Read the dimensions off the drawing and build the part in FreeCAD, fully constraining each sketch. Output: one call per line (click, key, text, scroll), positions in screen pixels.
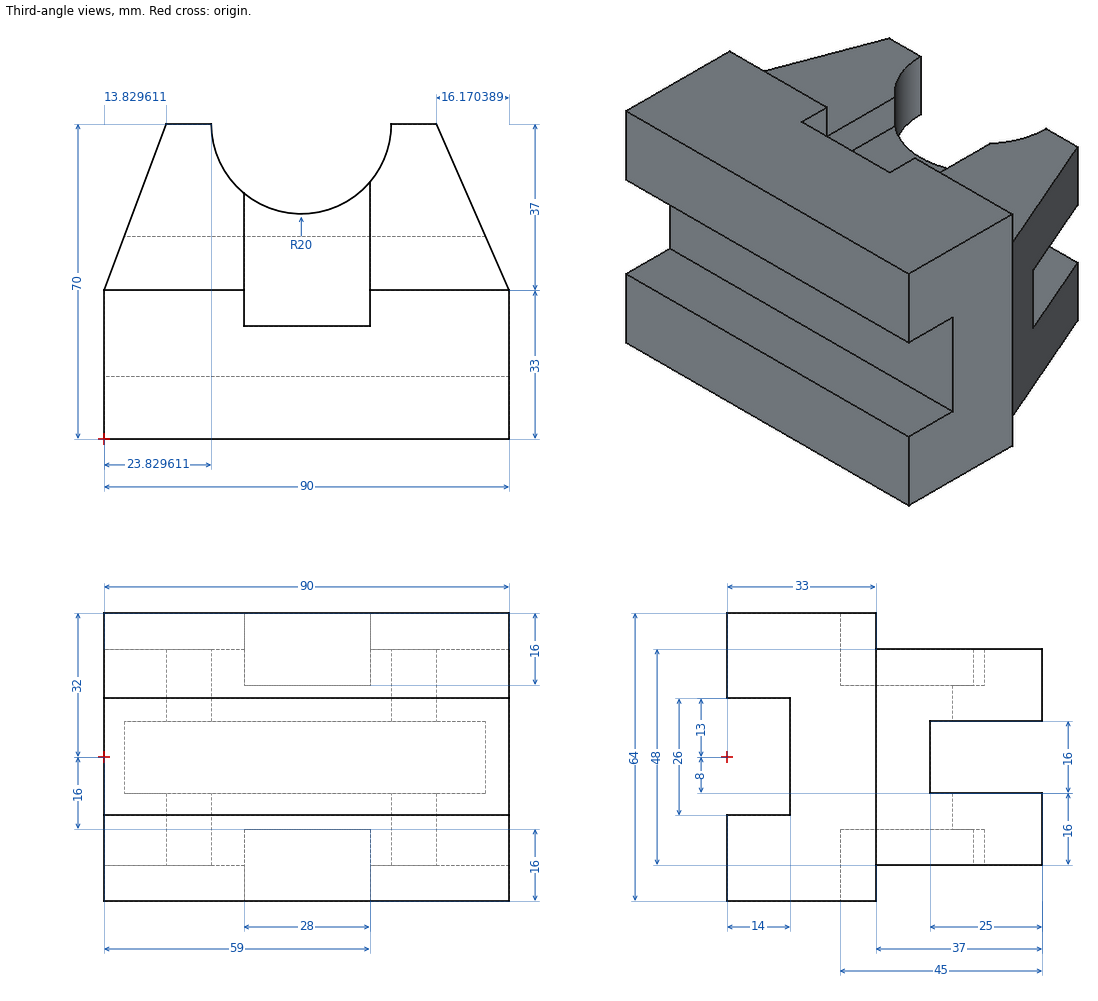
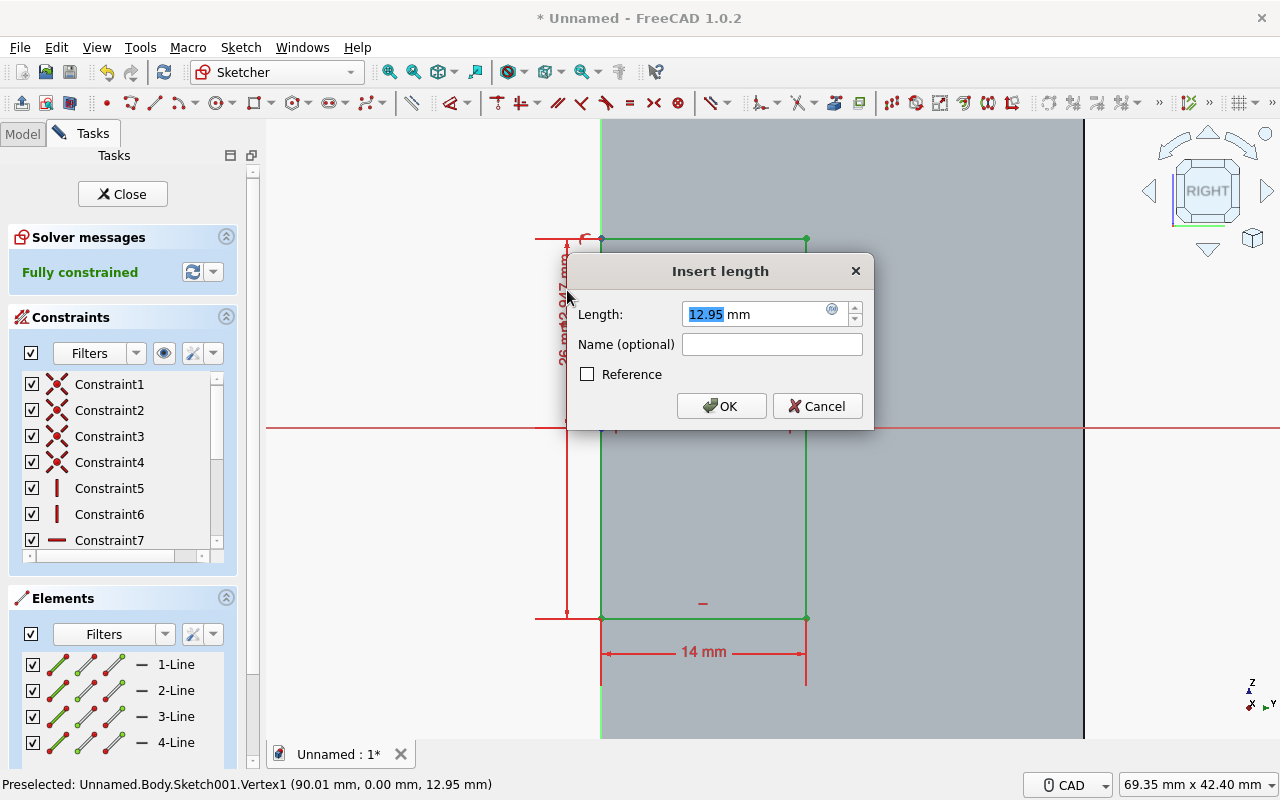
text(13)
key(Return)
key(Escape)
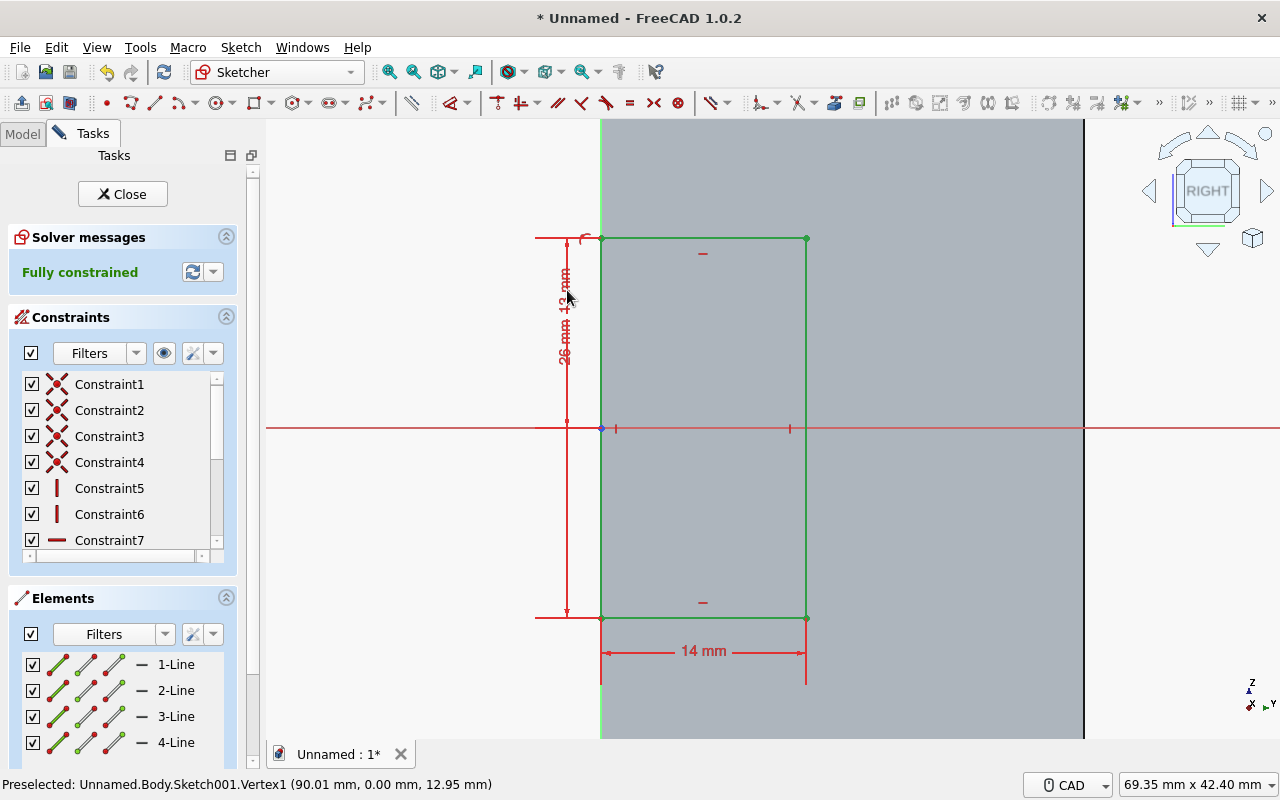
click(123, 194)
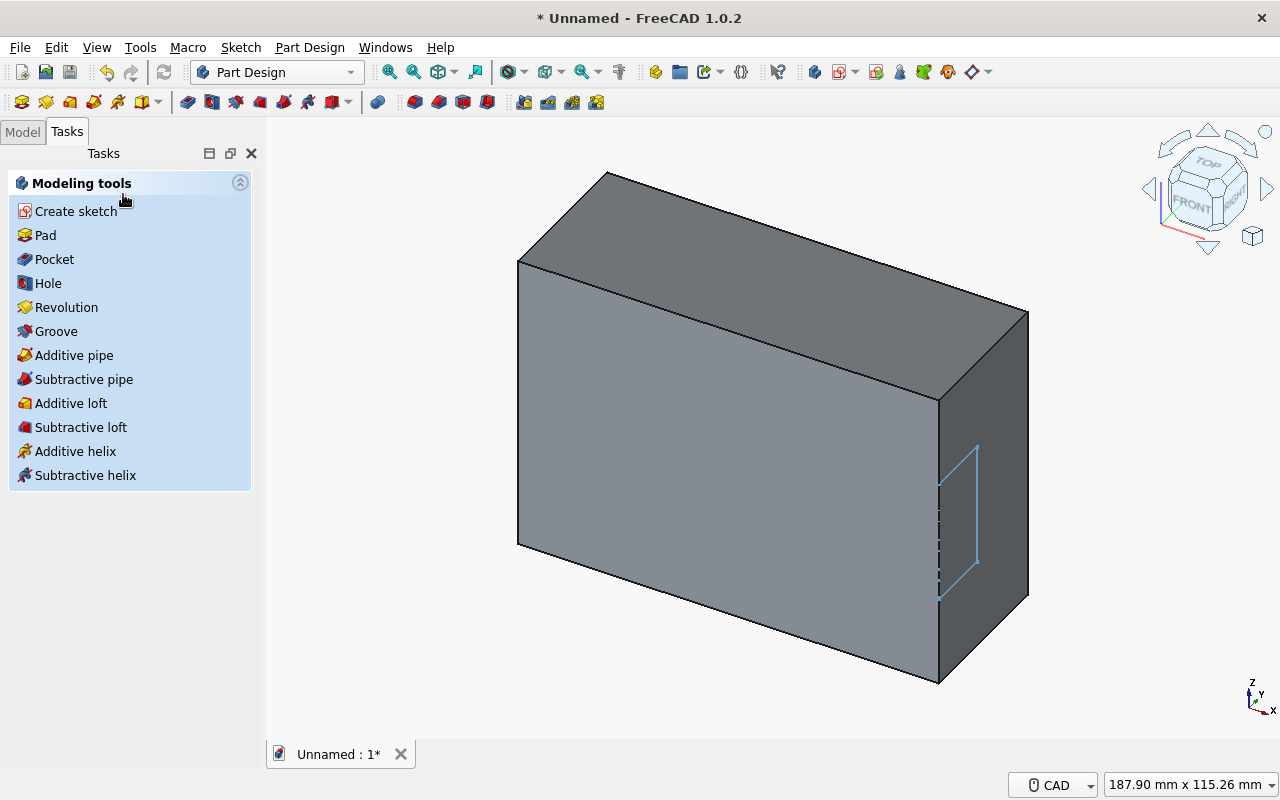
click(188, 102)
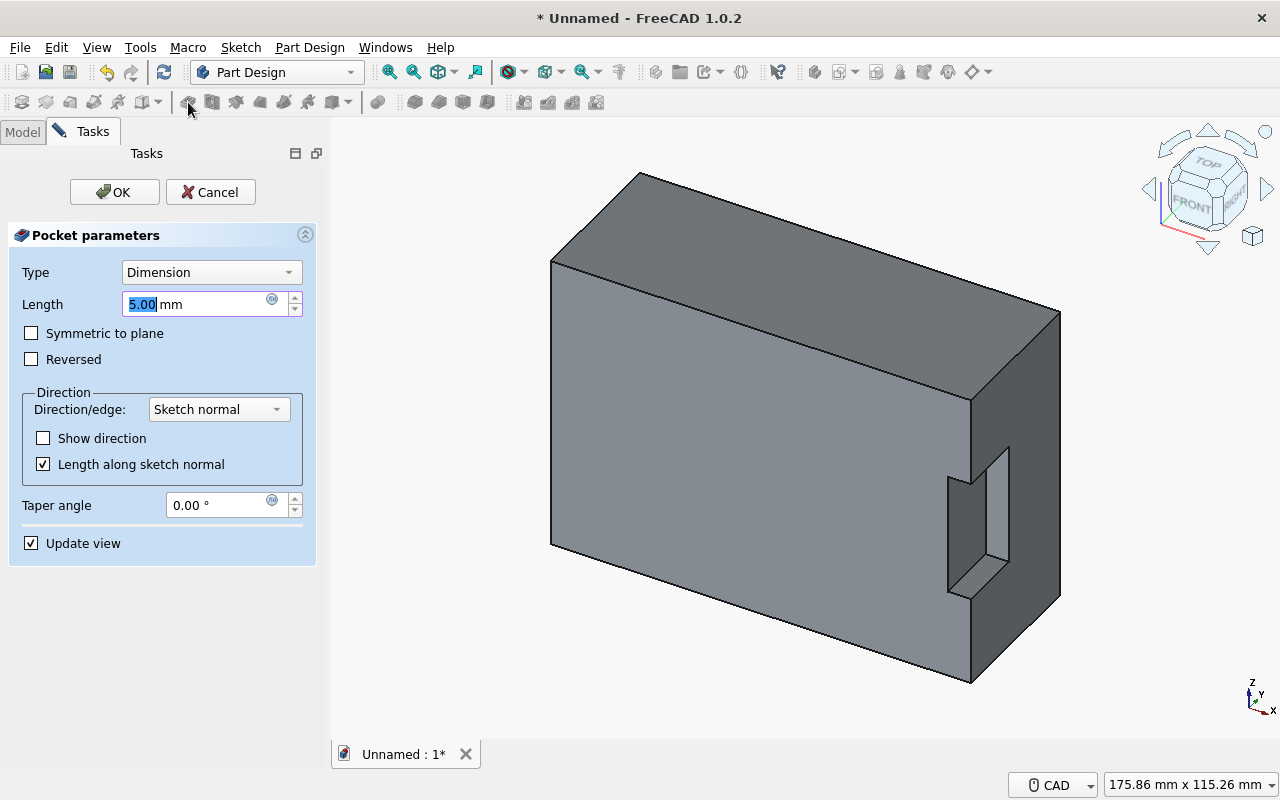
click(212, 272)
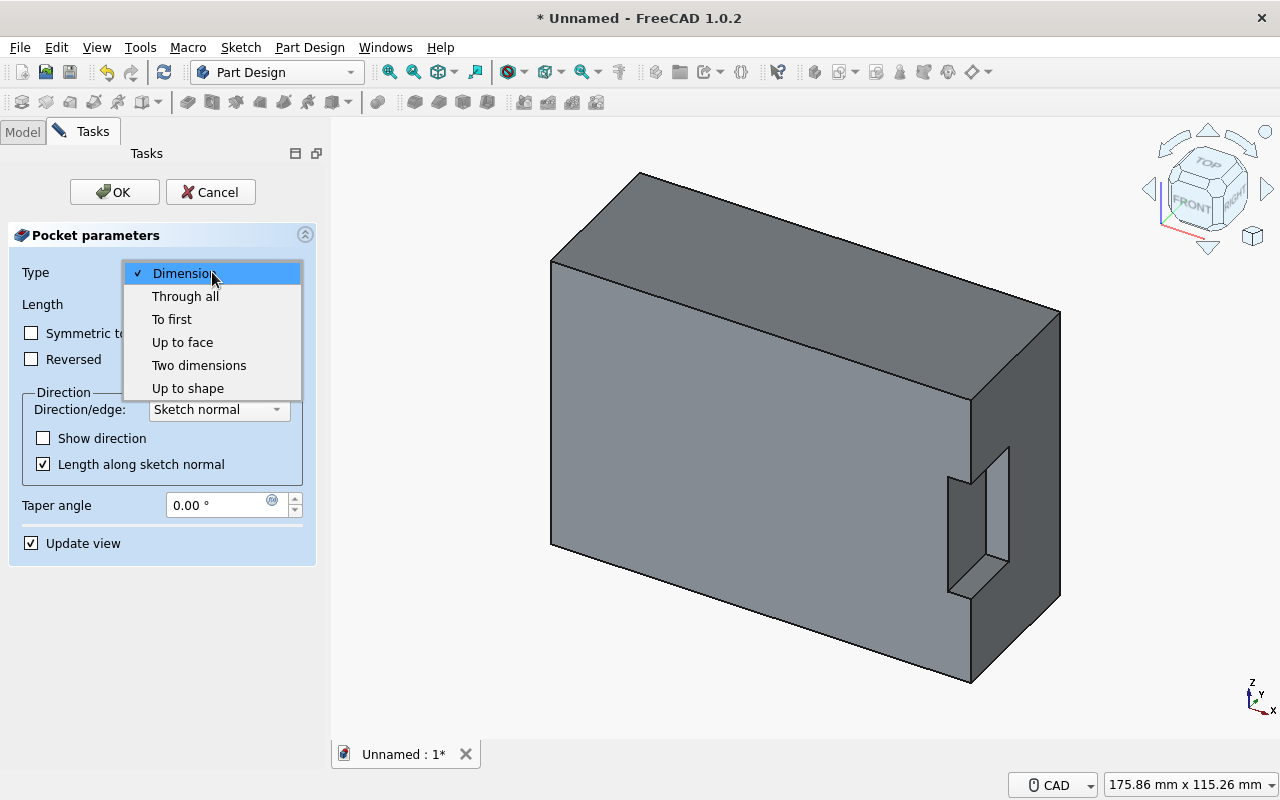
click(212, 296)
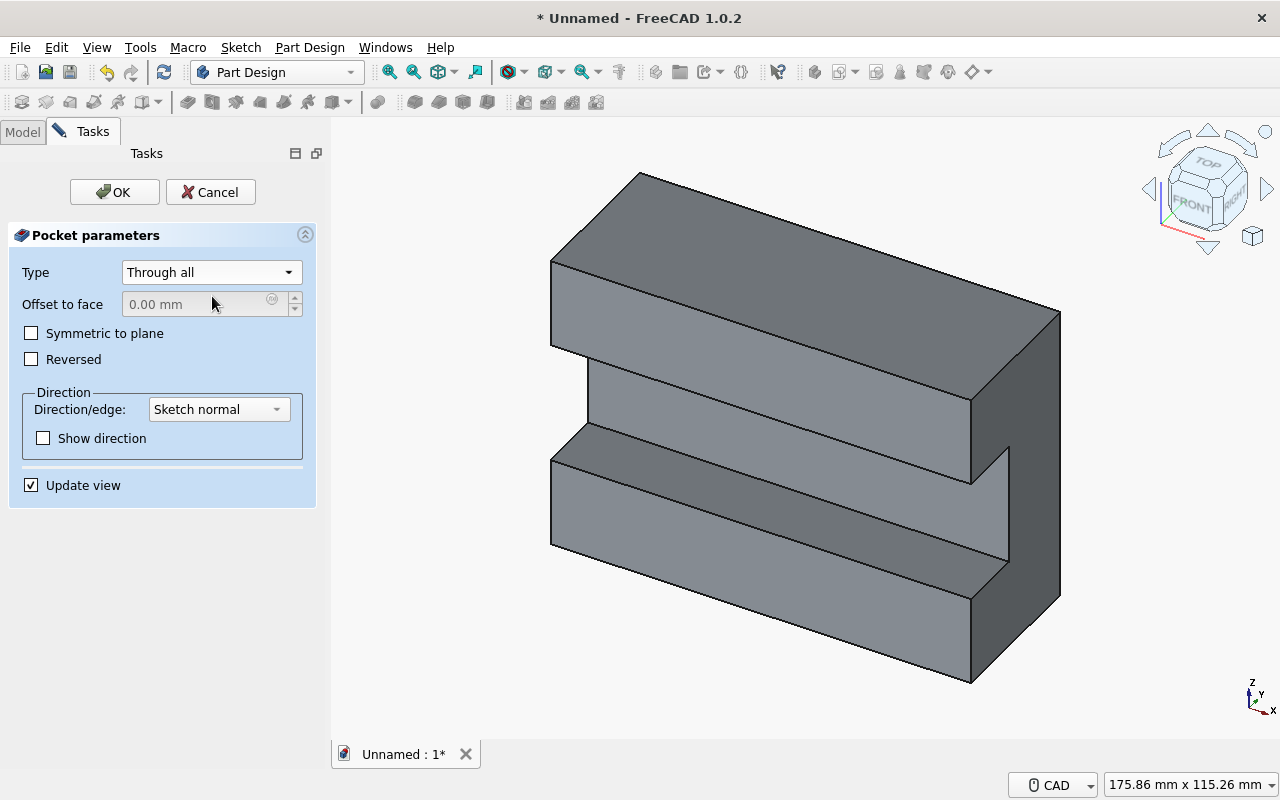
click(115, 192)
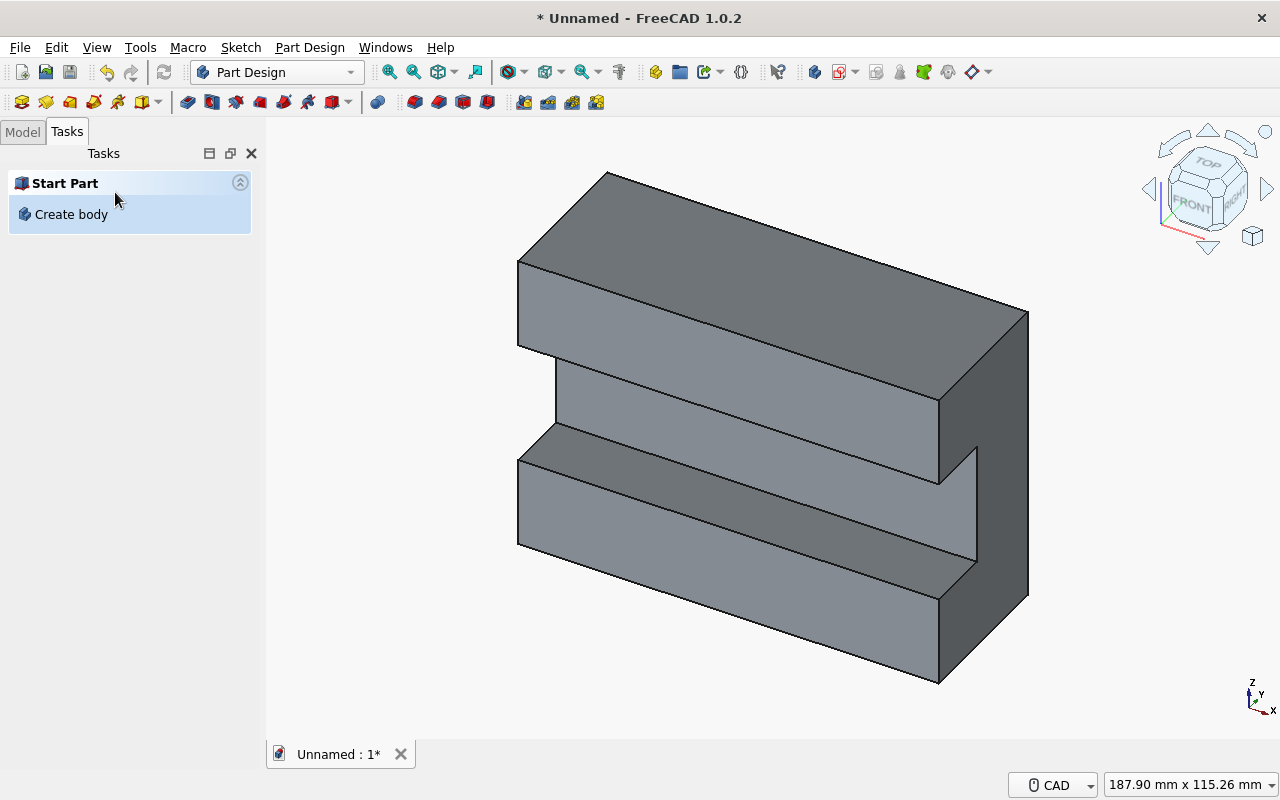
click(996, 403)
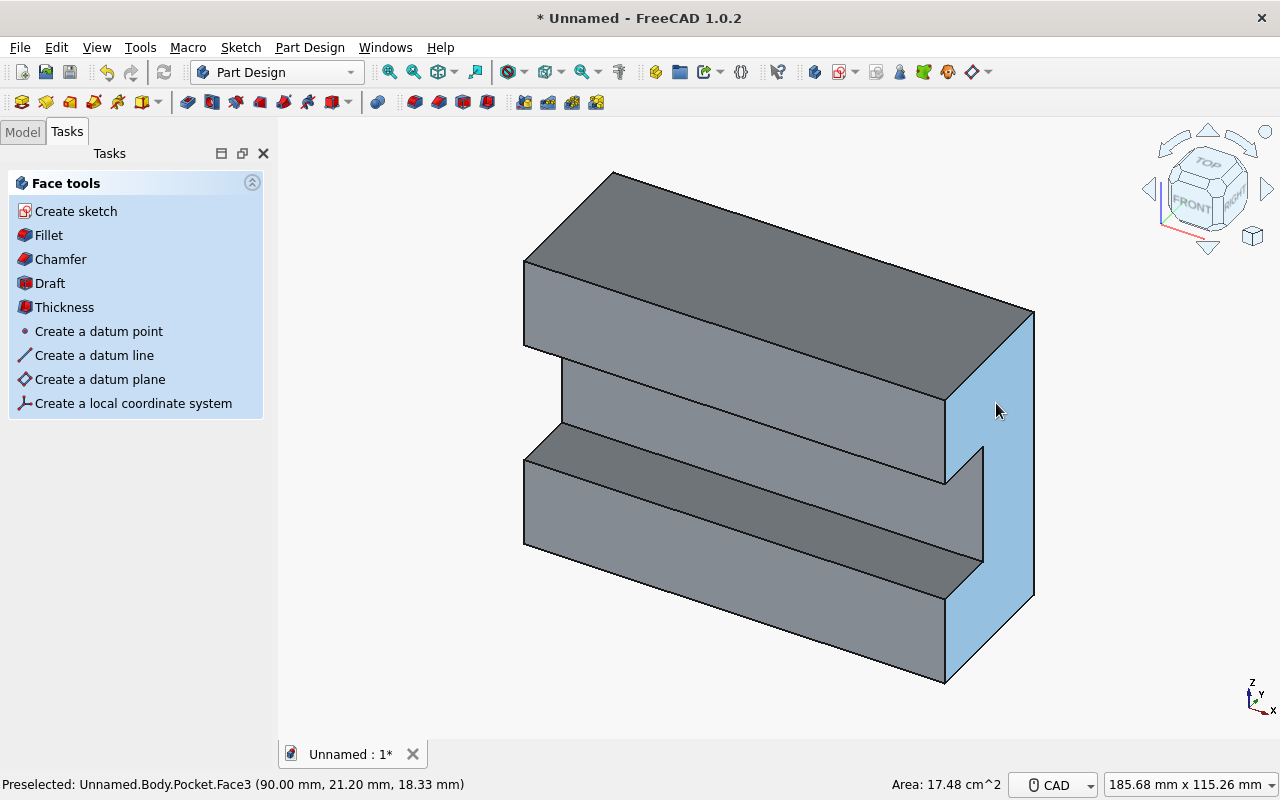
click(840, 72)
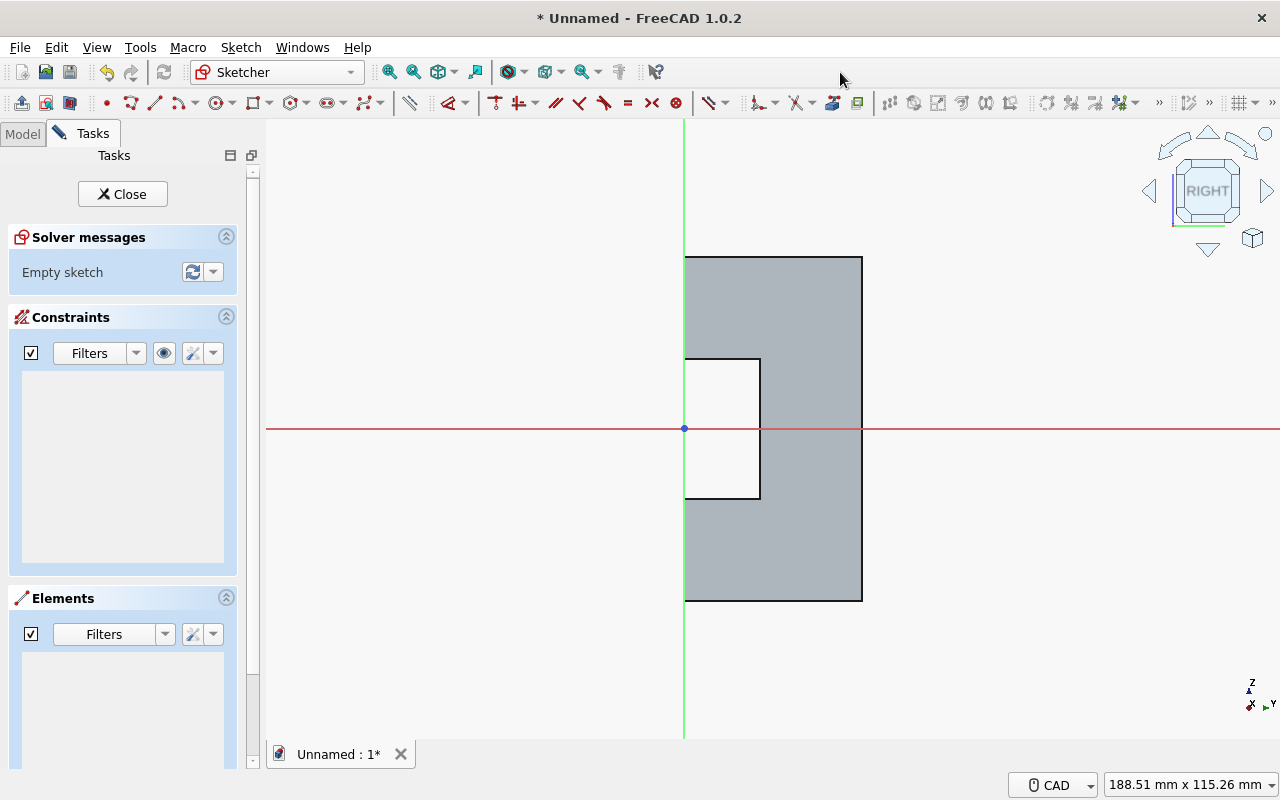
scroll(1115, 429, up, 2)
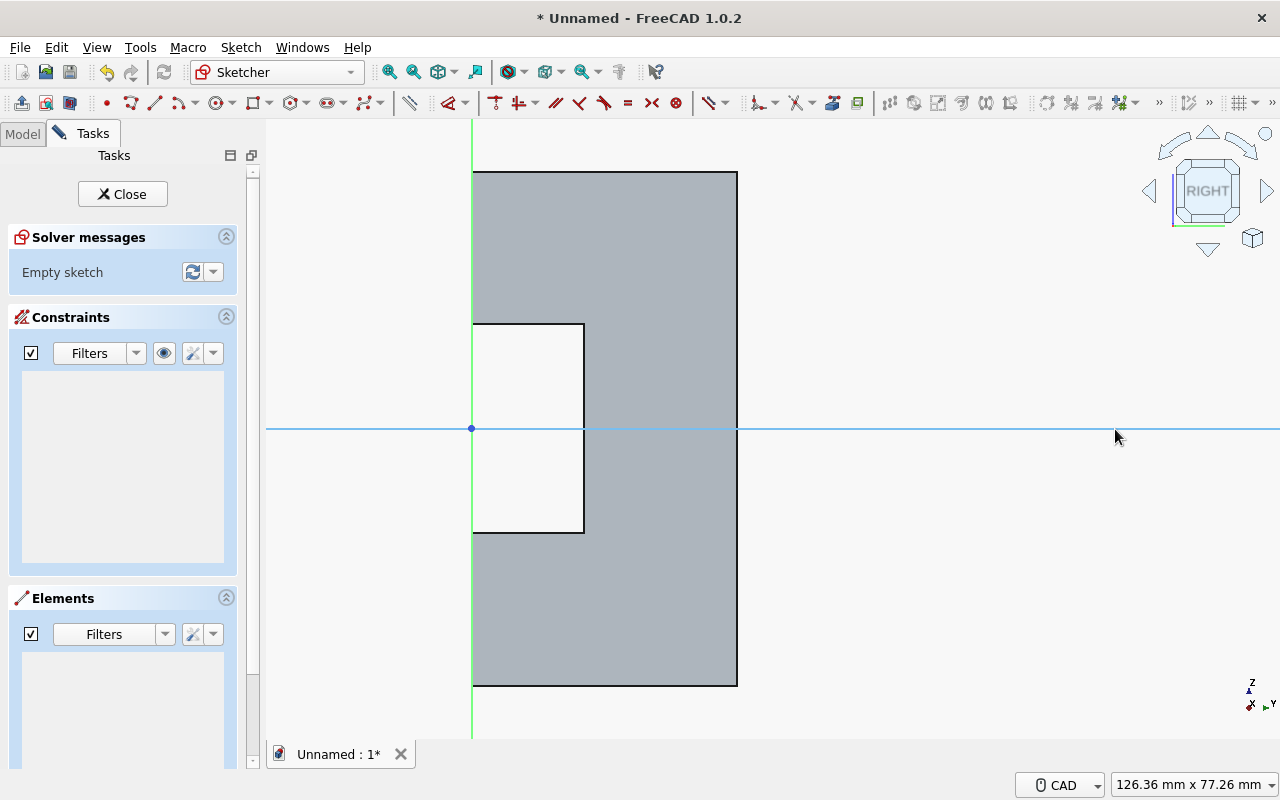
click(132, 104)